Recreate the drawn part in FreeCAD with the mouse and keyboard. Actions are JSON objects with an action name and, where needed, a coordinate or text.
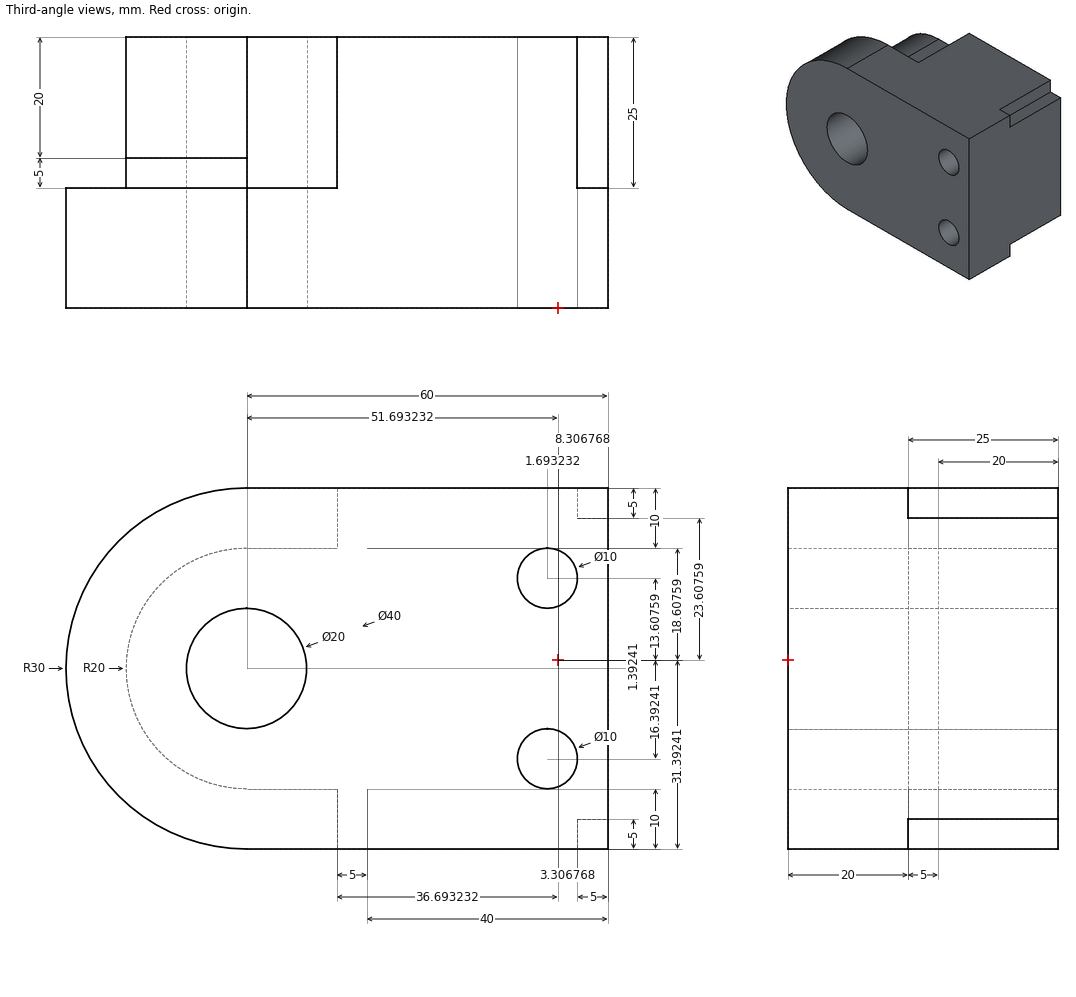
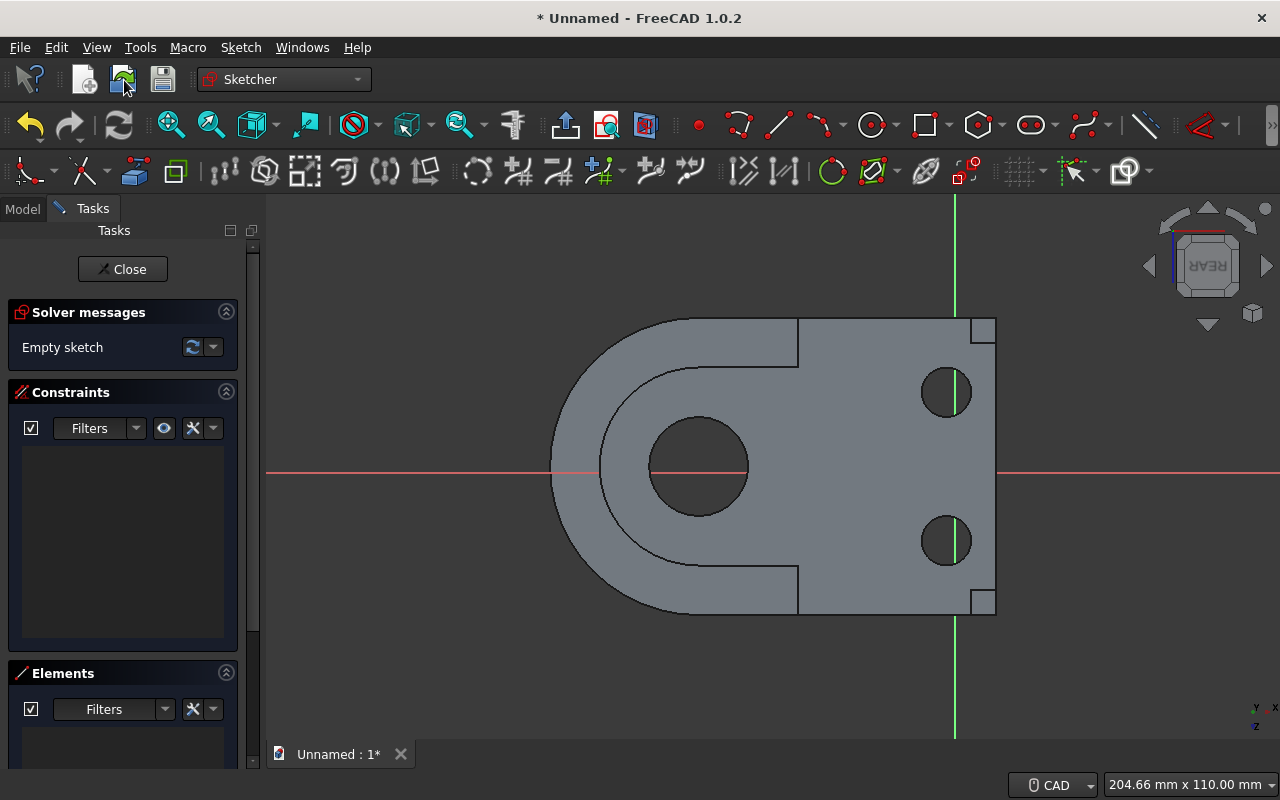
{"action": "key", "text": "q s"}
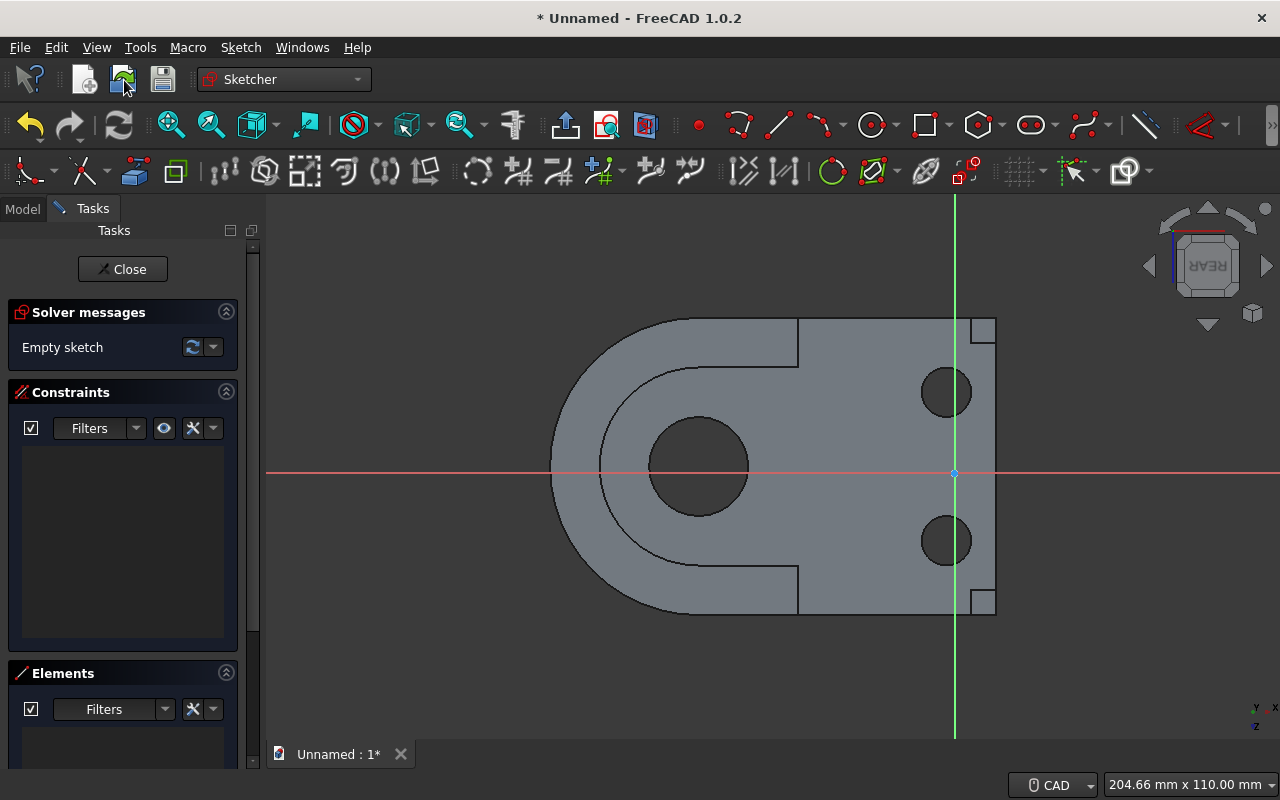
{"action": "key", "text": "g r"}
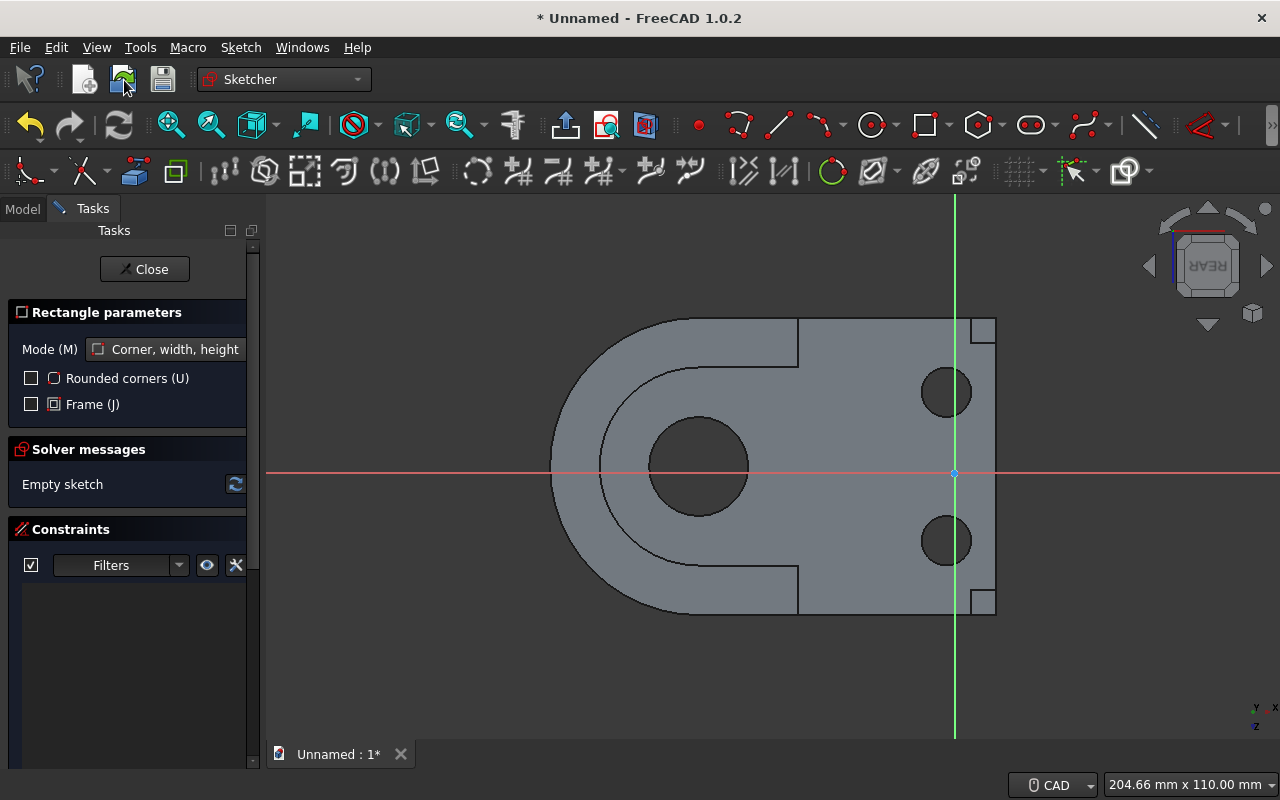
{"action": "left_click", "coordinate": [773, 318]}
{"action": "left_click", "coordinate": [798, 367]}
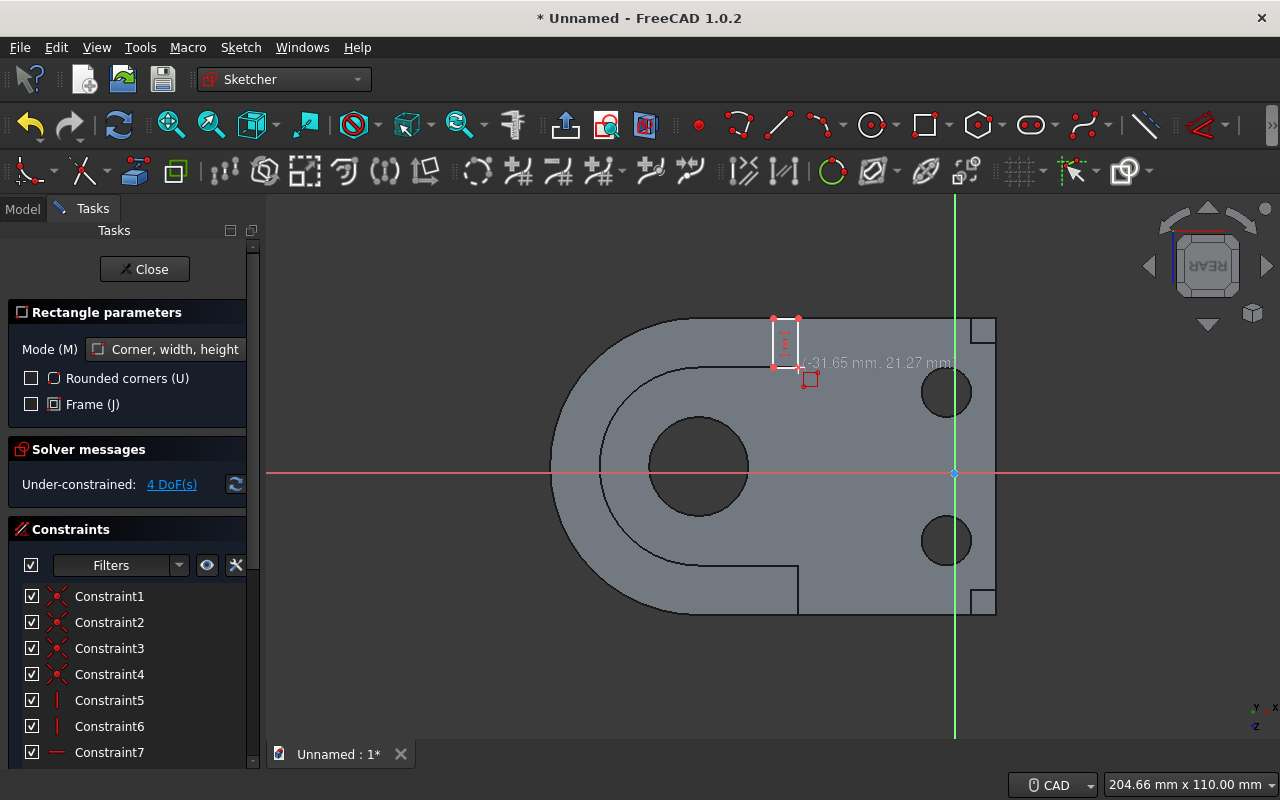
{"action": "left_click", "coordinate": [773, 566]}
{"action": "left_click", "coordinate": [798, 615]}
{"action": "key", "text": "Escape"}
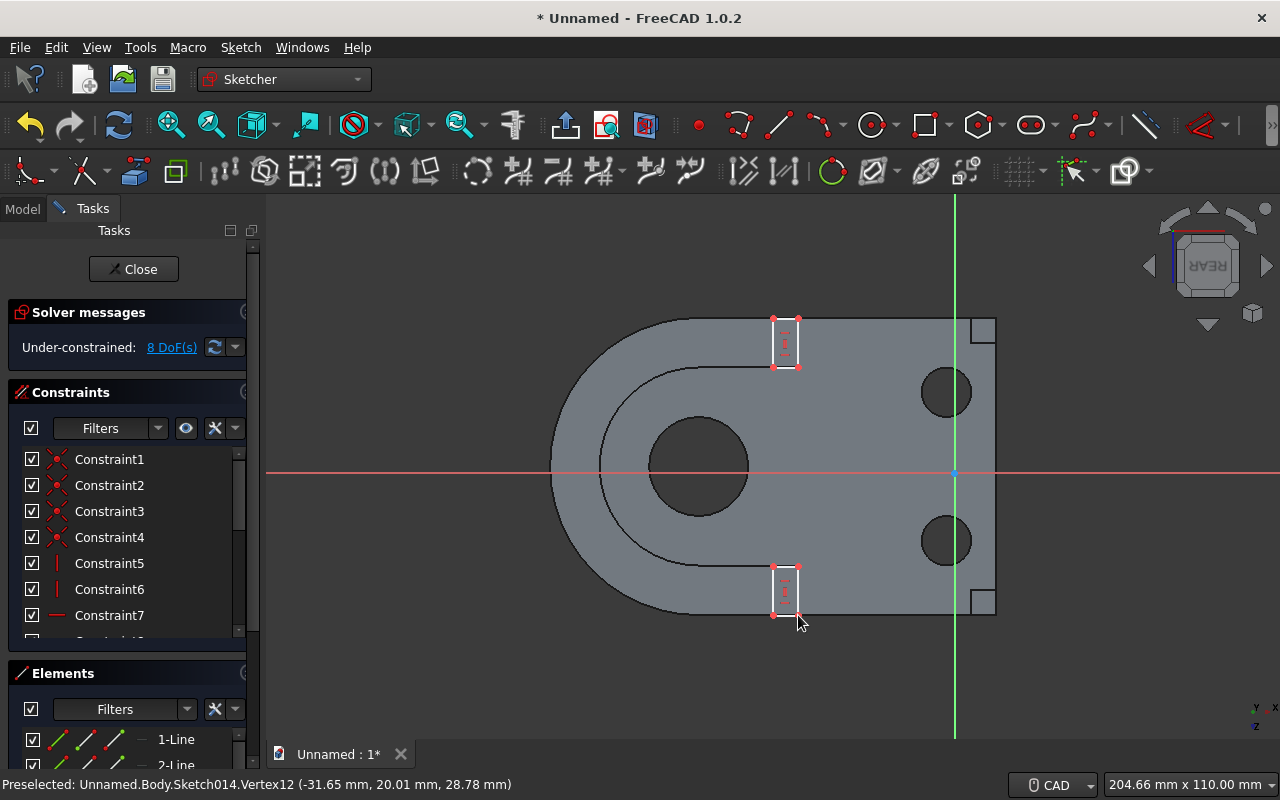
{"action": "left_click", "coordinate": [1200, 126]}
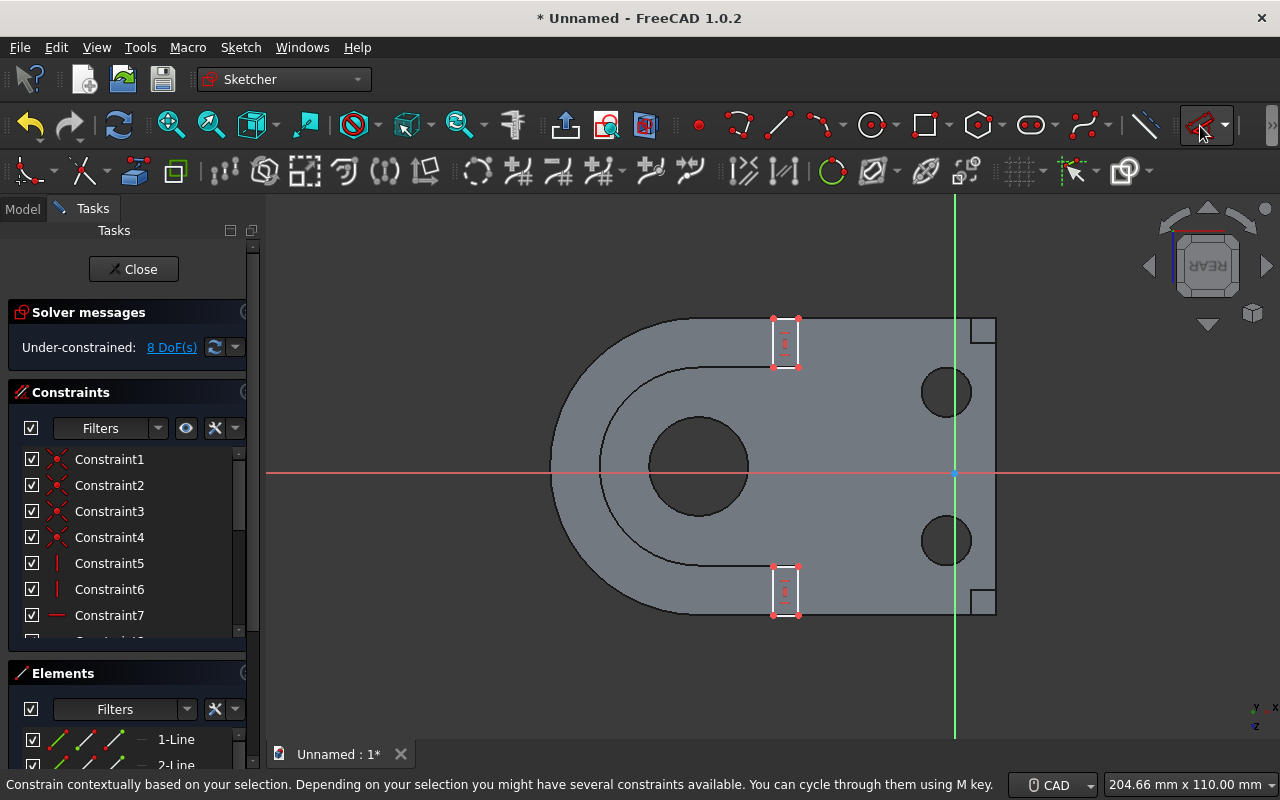
{"action": "scroll", "coordinate": [783, 368], "scroll_direction": "up", "scroll_amount": 3}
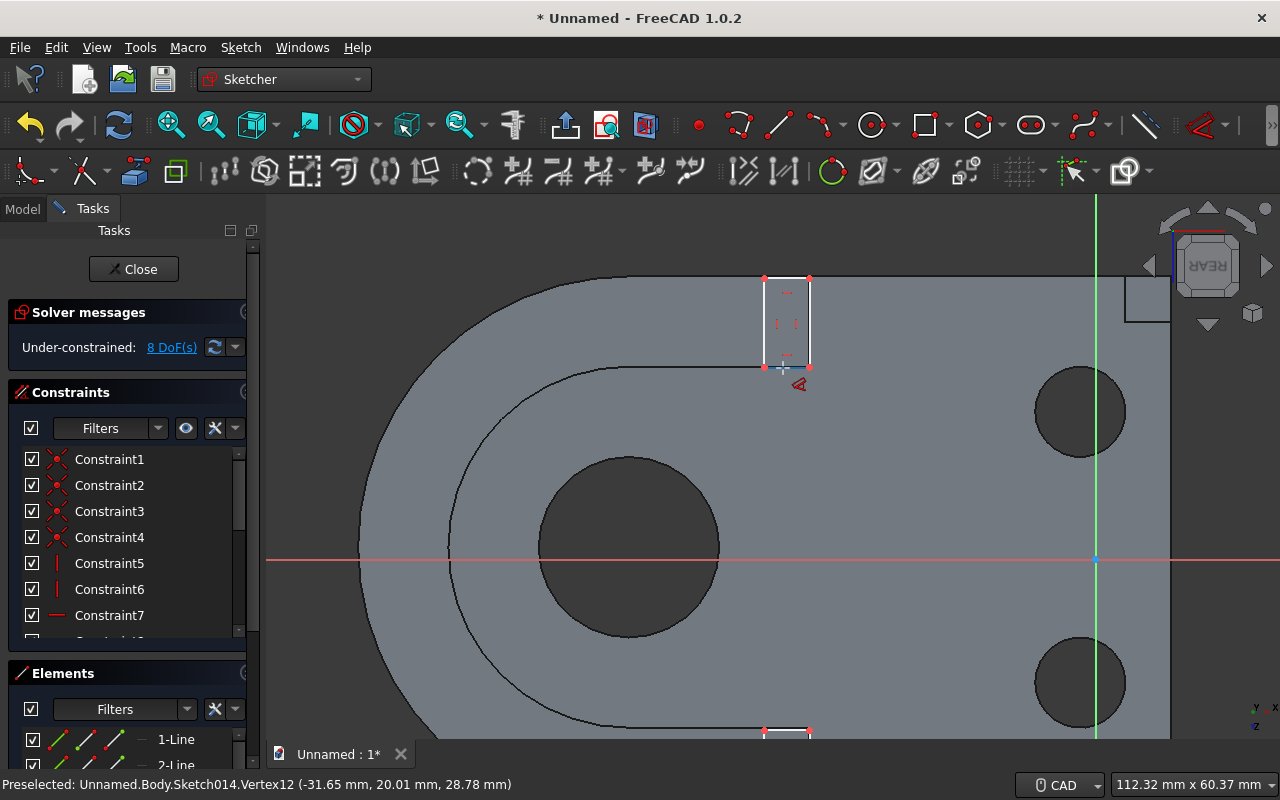
{"action": "left_click", "coordinate": [783, 368]}
{"action": "left_click", "coordinate": [787, 334]}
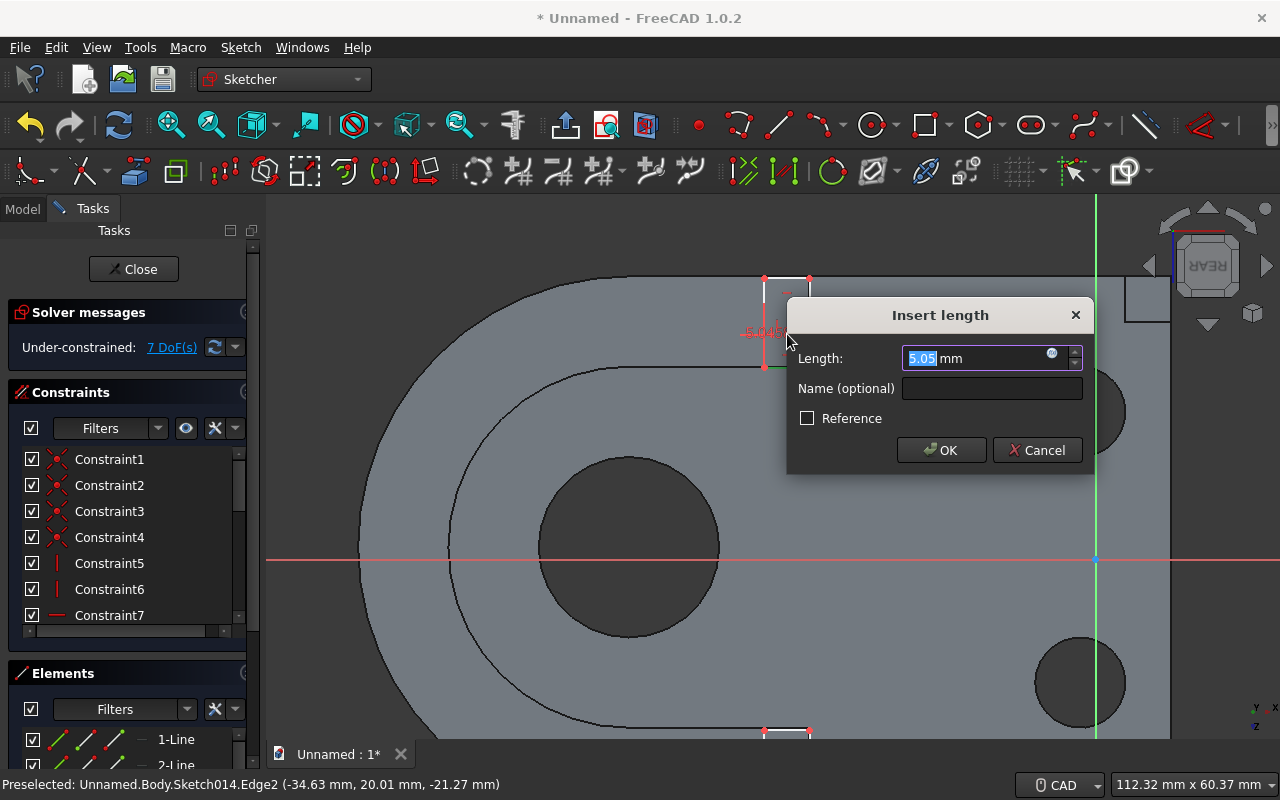
{"action": "type", "text": "5"}
{"action": "key", "text": "Return"}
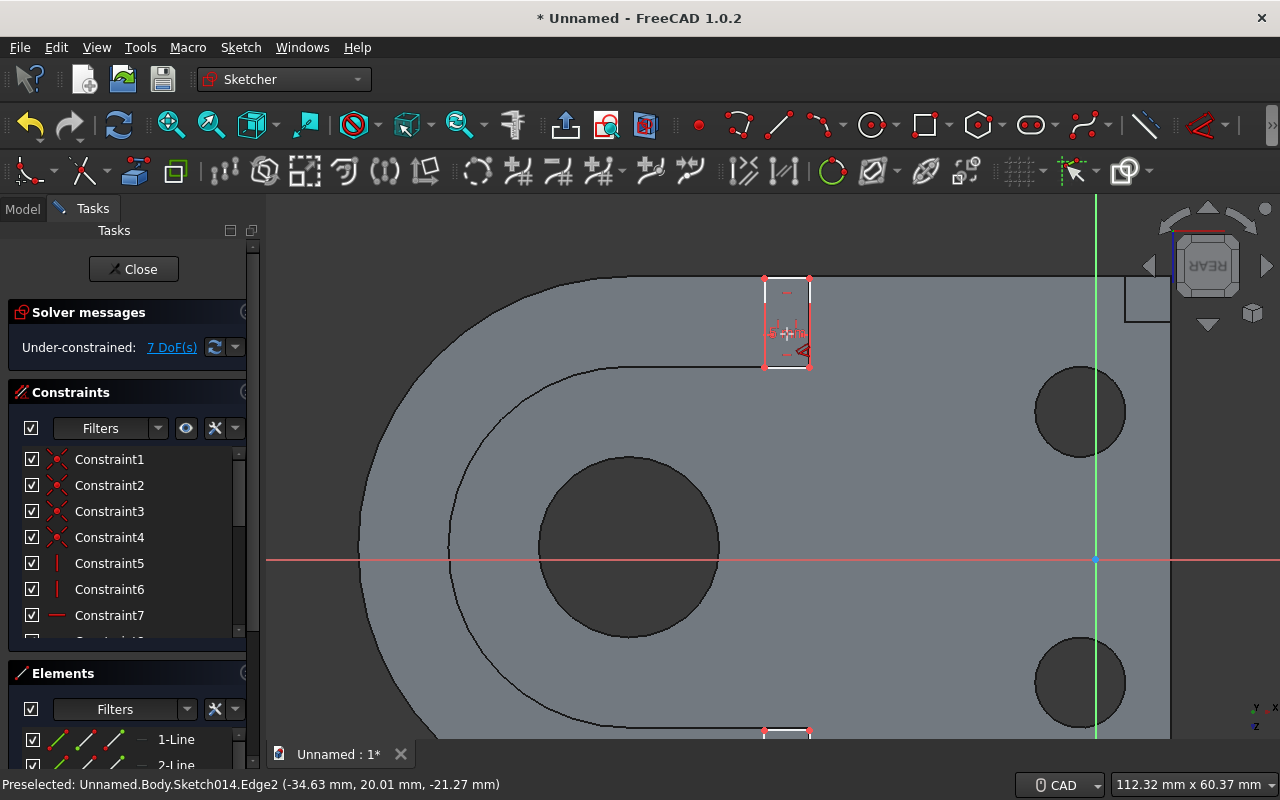
{"action": "scroll", "coordinate": [294, 302], "scroll_direction": "down", "scroll_amount": 2}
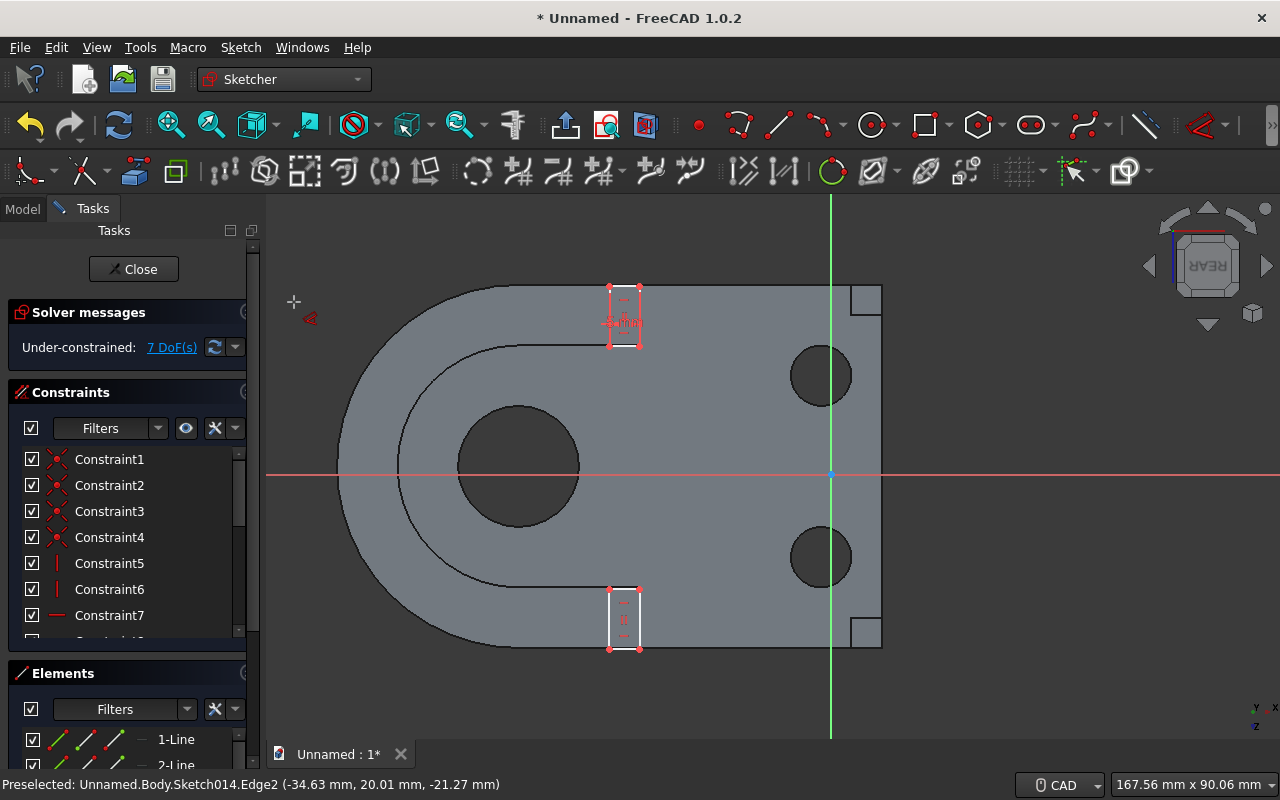
{"action": "scroll", "coordinate": [618, 649], "scroll_direction": "up", "scroll_amount": 3}